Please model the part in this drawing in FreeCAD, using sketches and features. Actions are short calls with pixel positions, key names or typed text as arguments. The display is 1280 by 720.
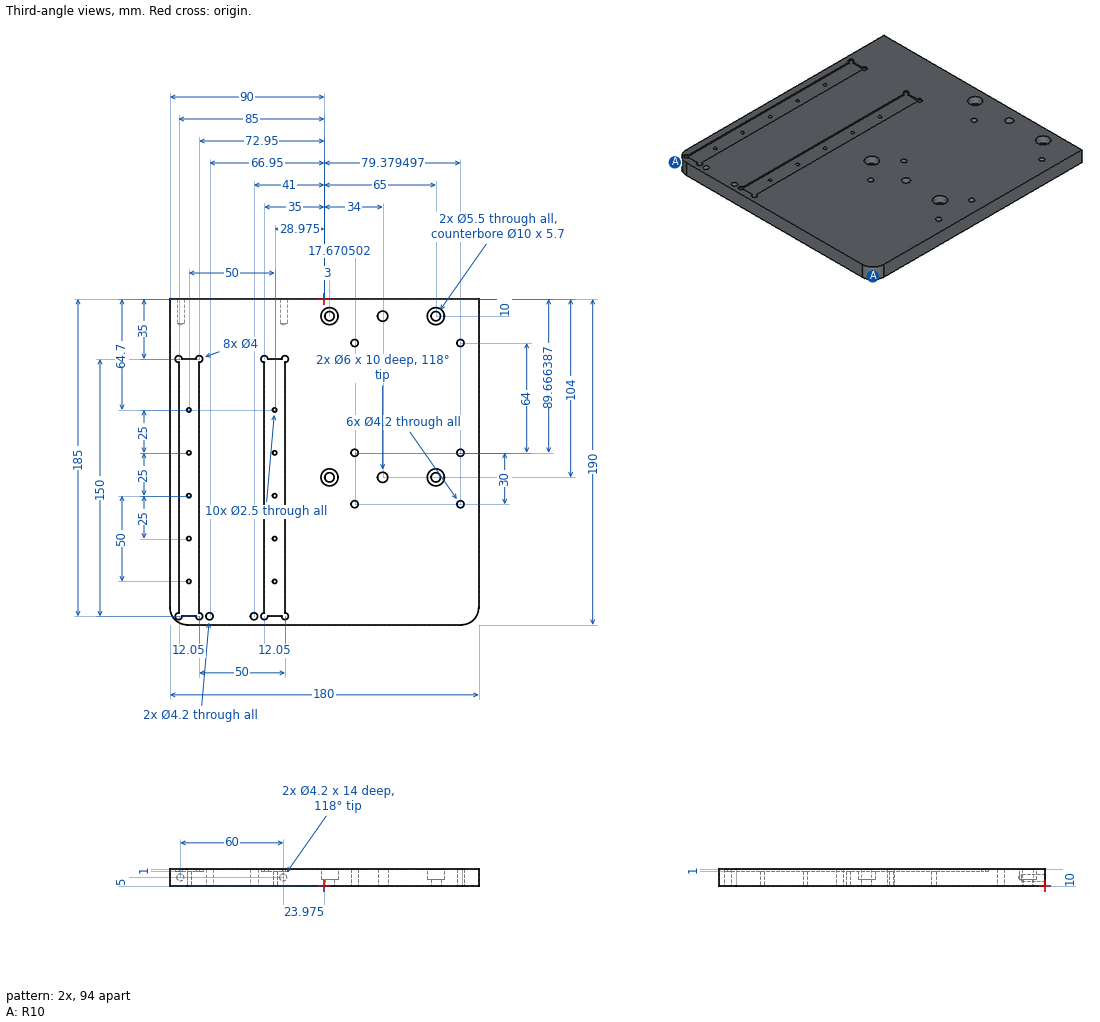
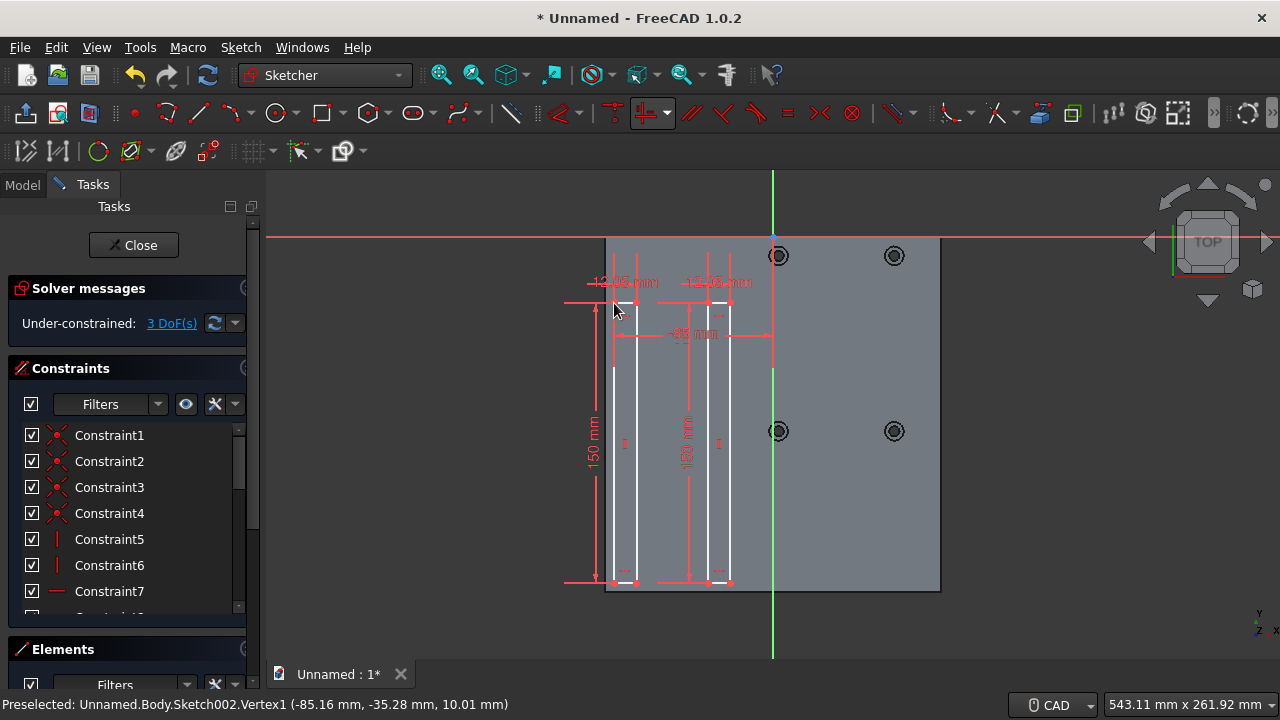
click(614, 303)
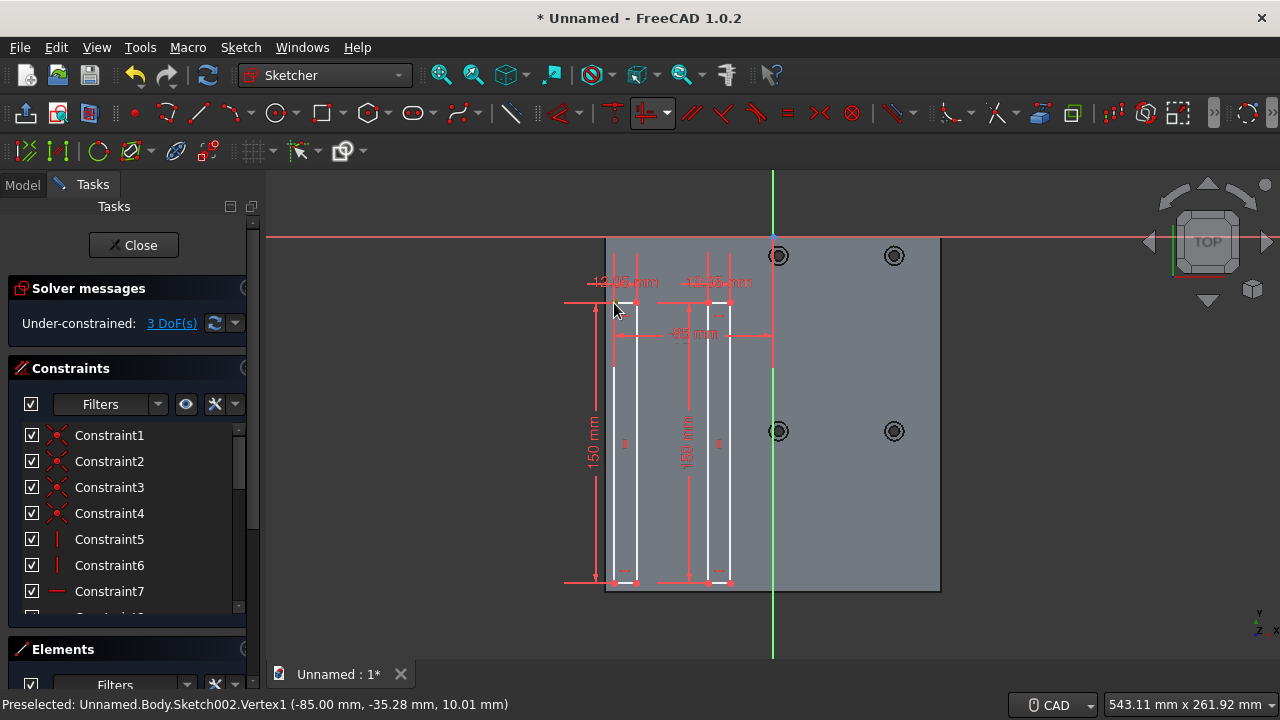
key(i)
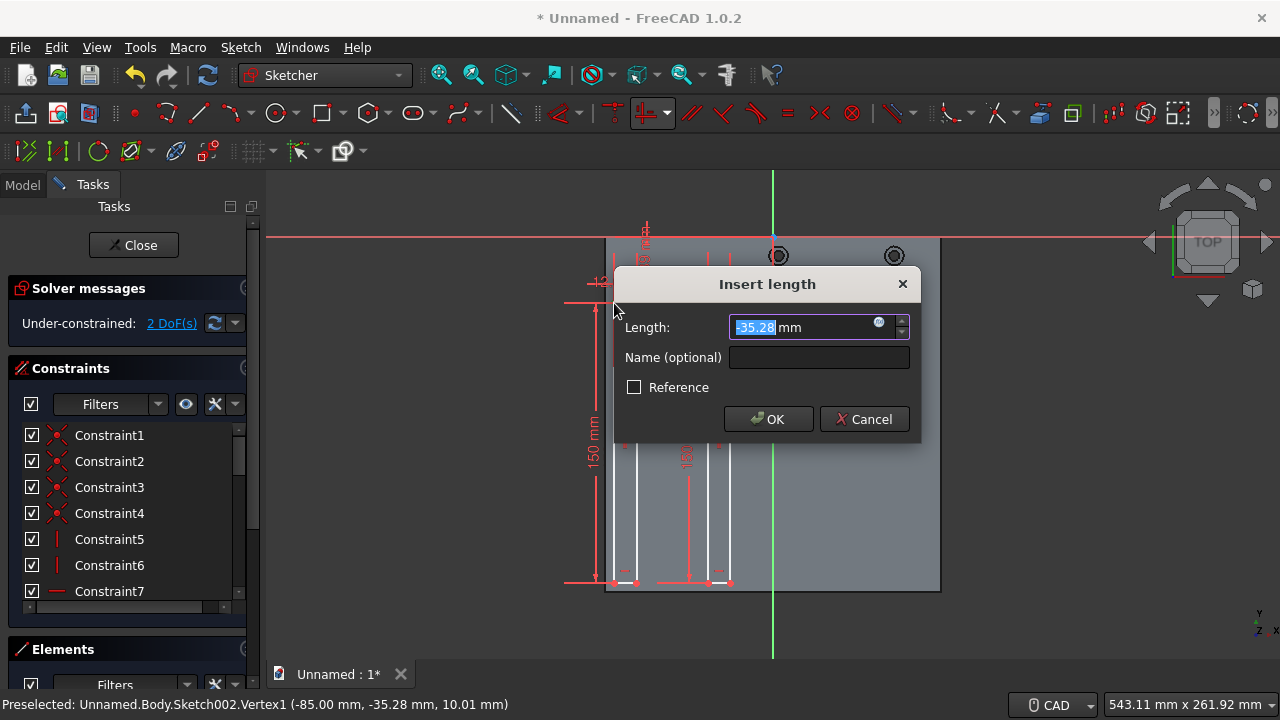
text(-35)
key(Return)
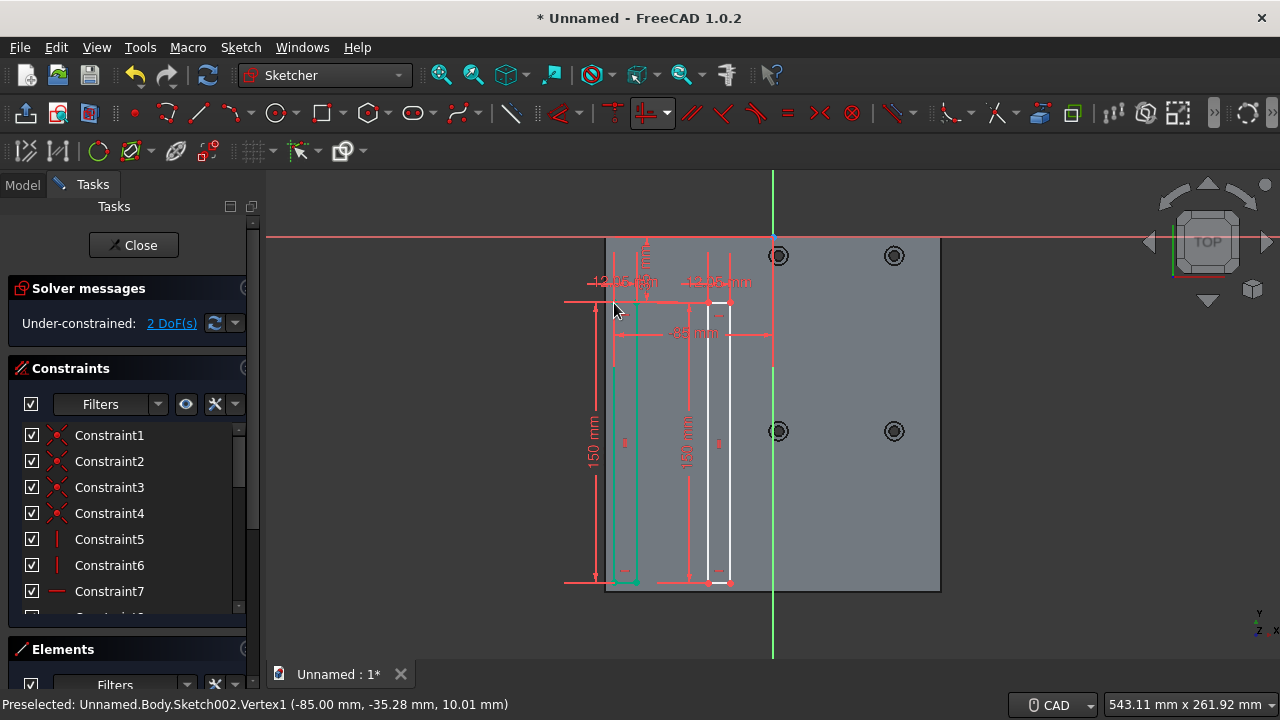
click(708, 303)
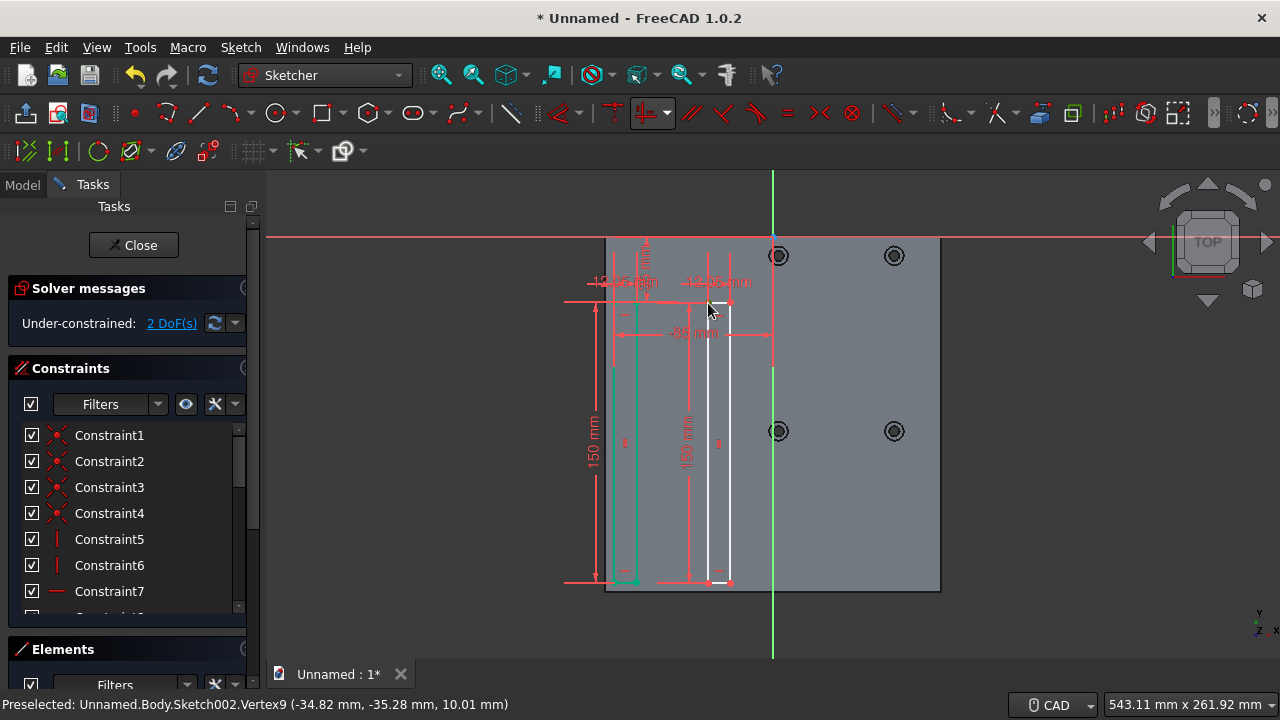
key(l)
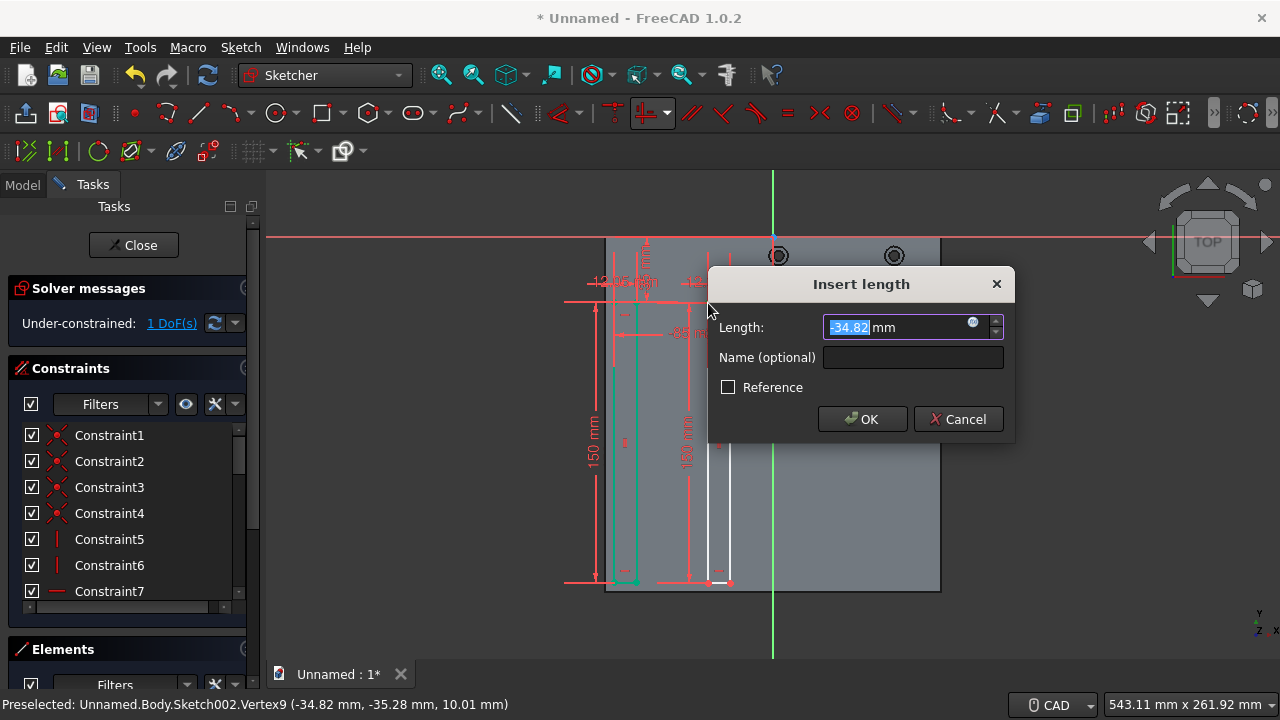
text(-35)
key(Return)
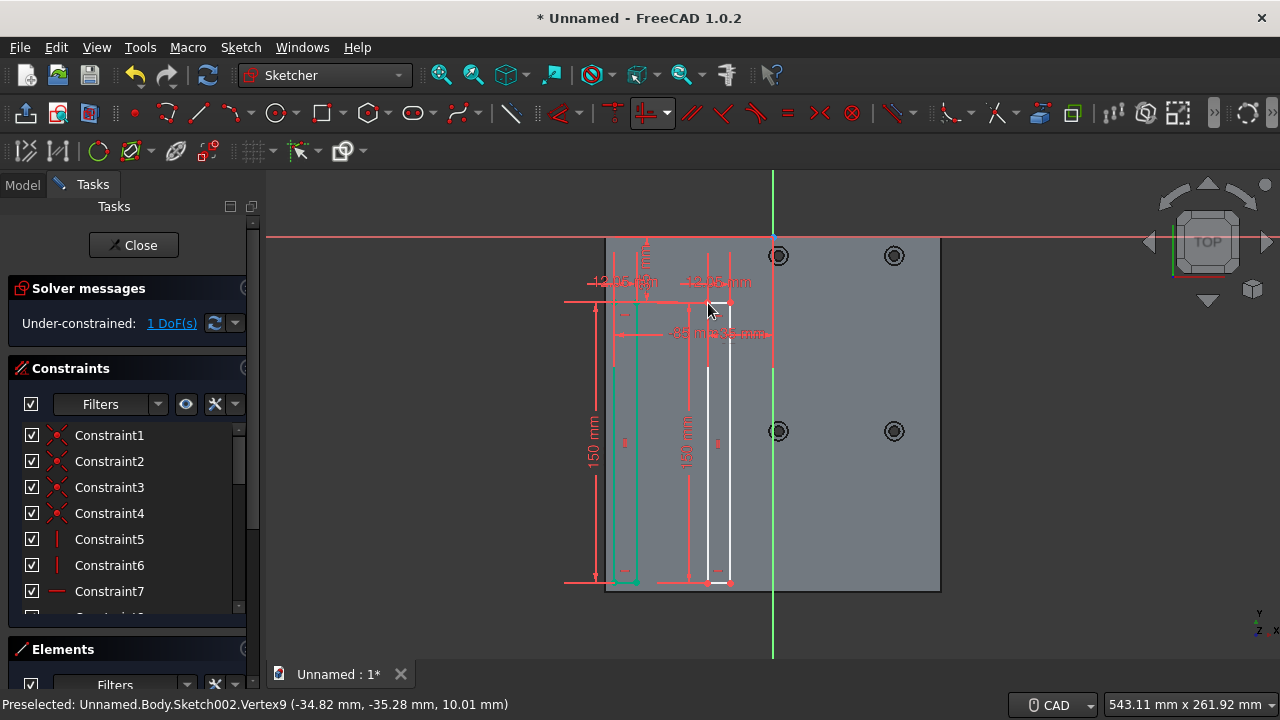
click(708, 303)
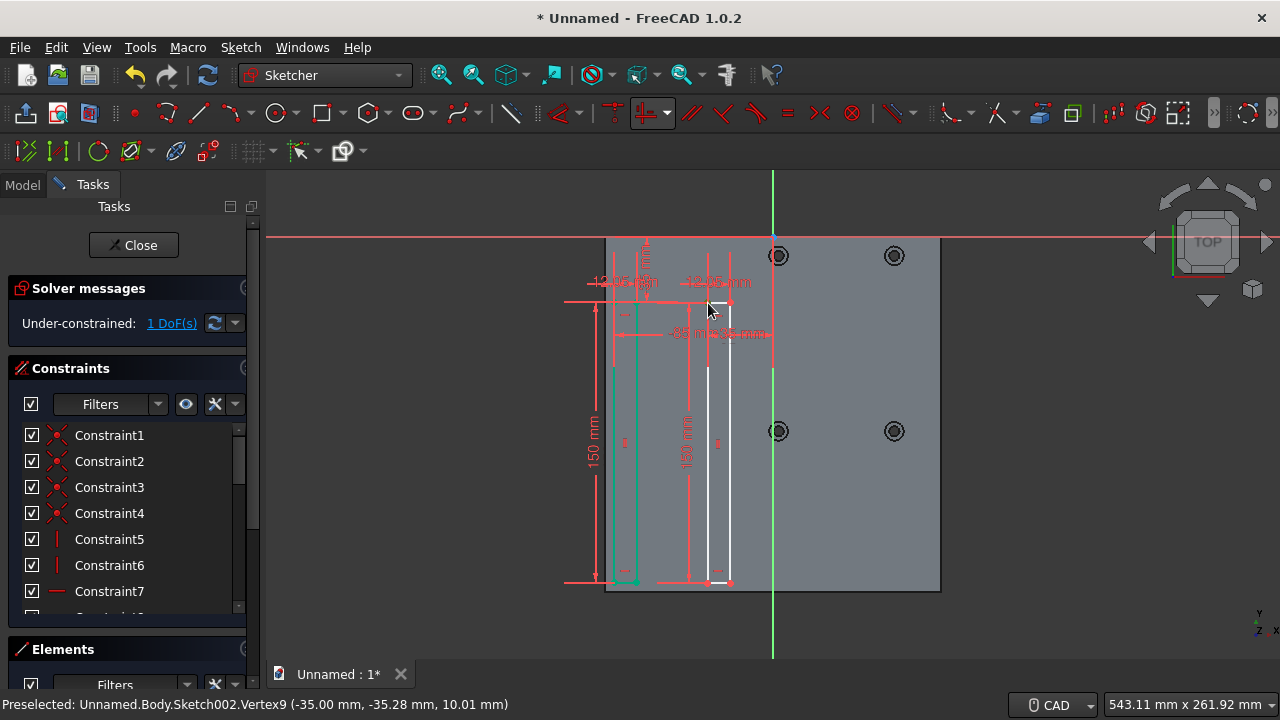
key(i)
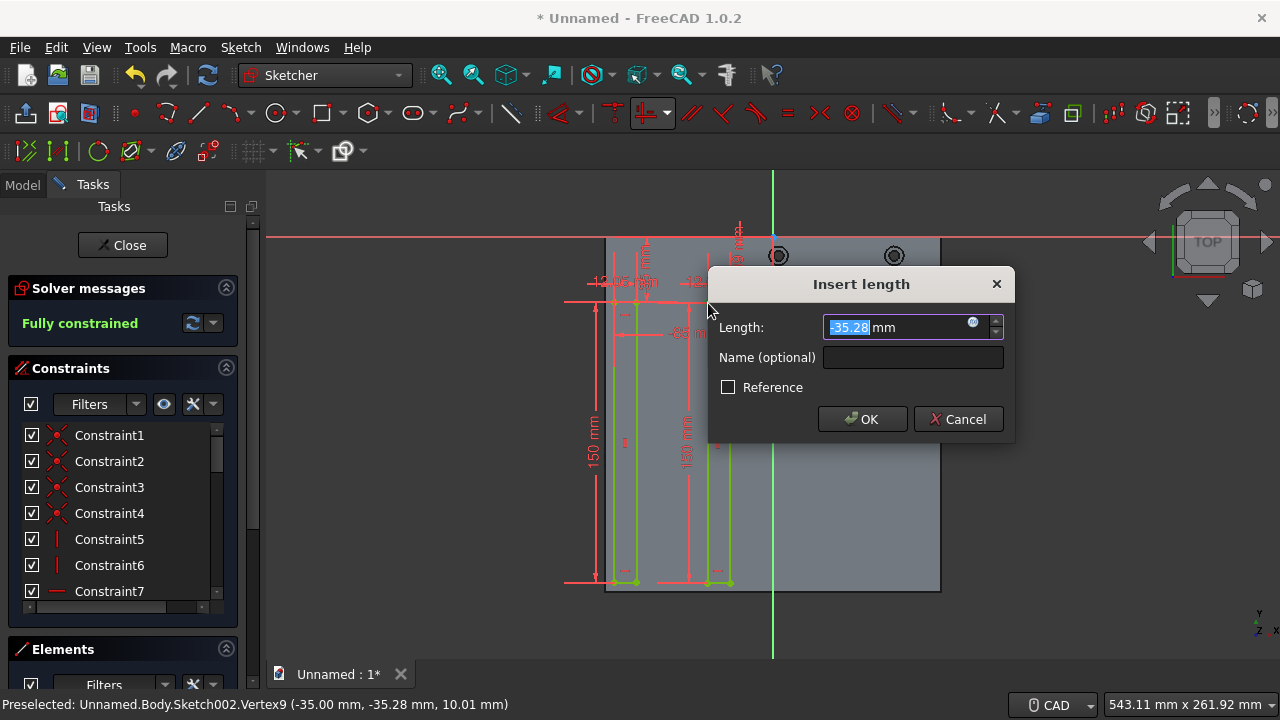
text(-35)
key(Return)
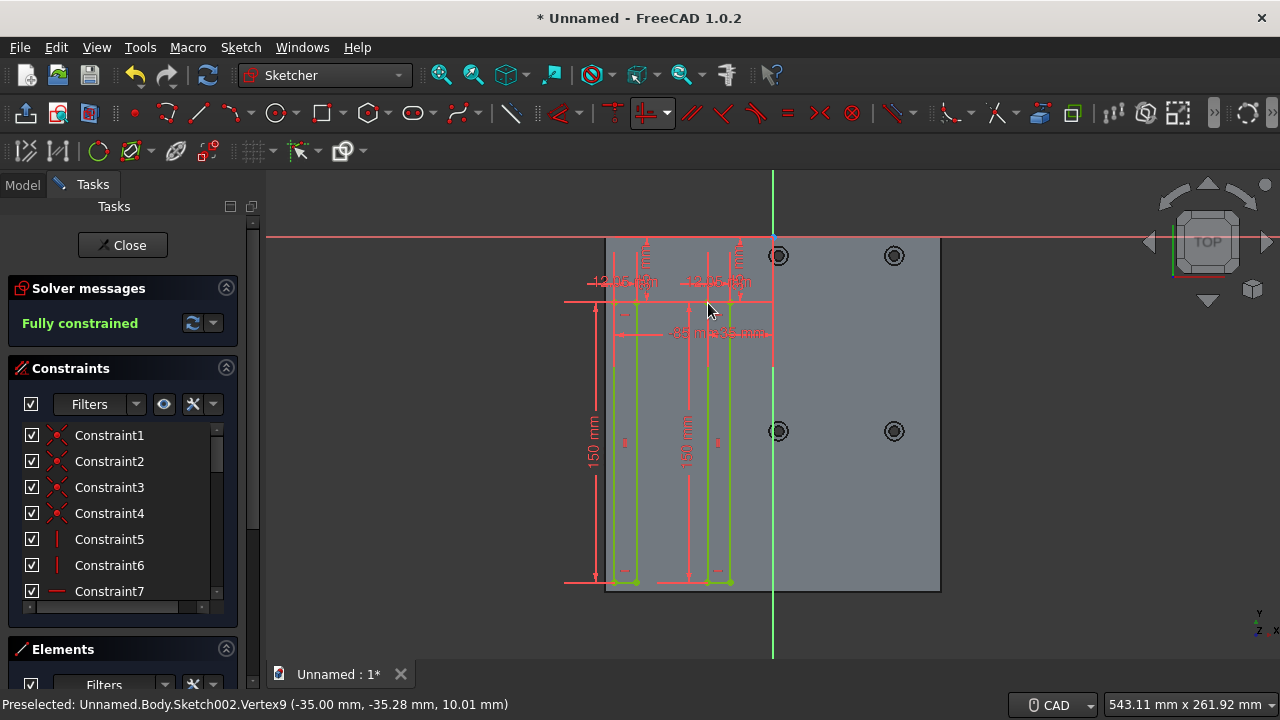
click(123, 245)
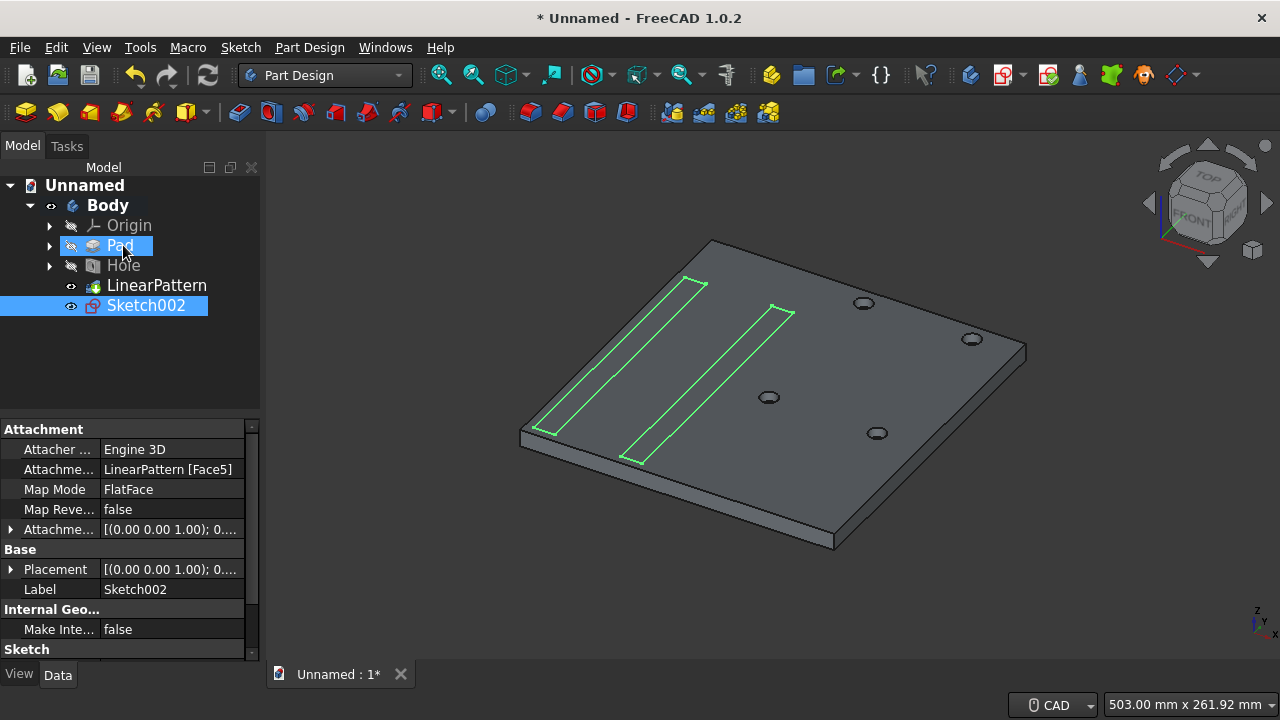
click(240, 112)